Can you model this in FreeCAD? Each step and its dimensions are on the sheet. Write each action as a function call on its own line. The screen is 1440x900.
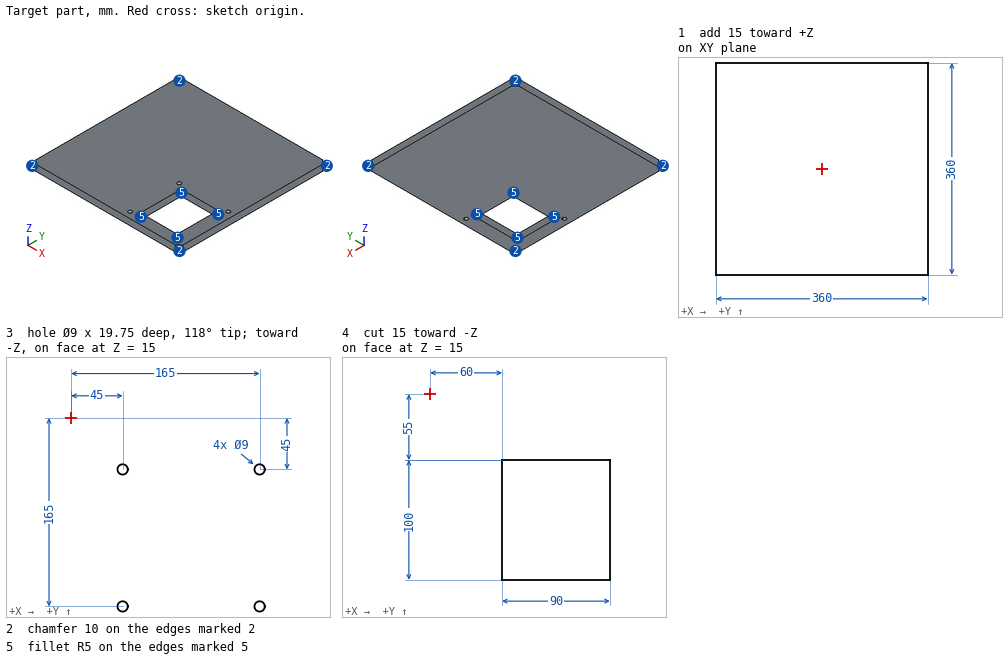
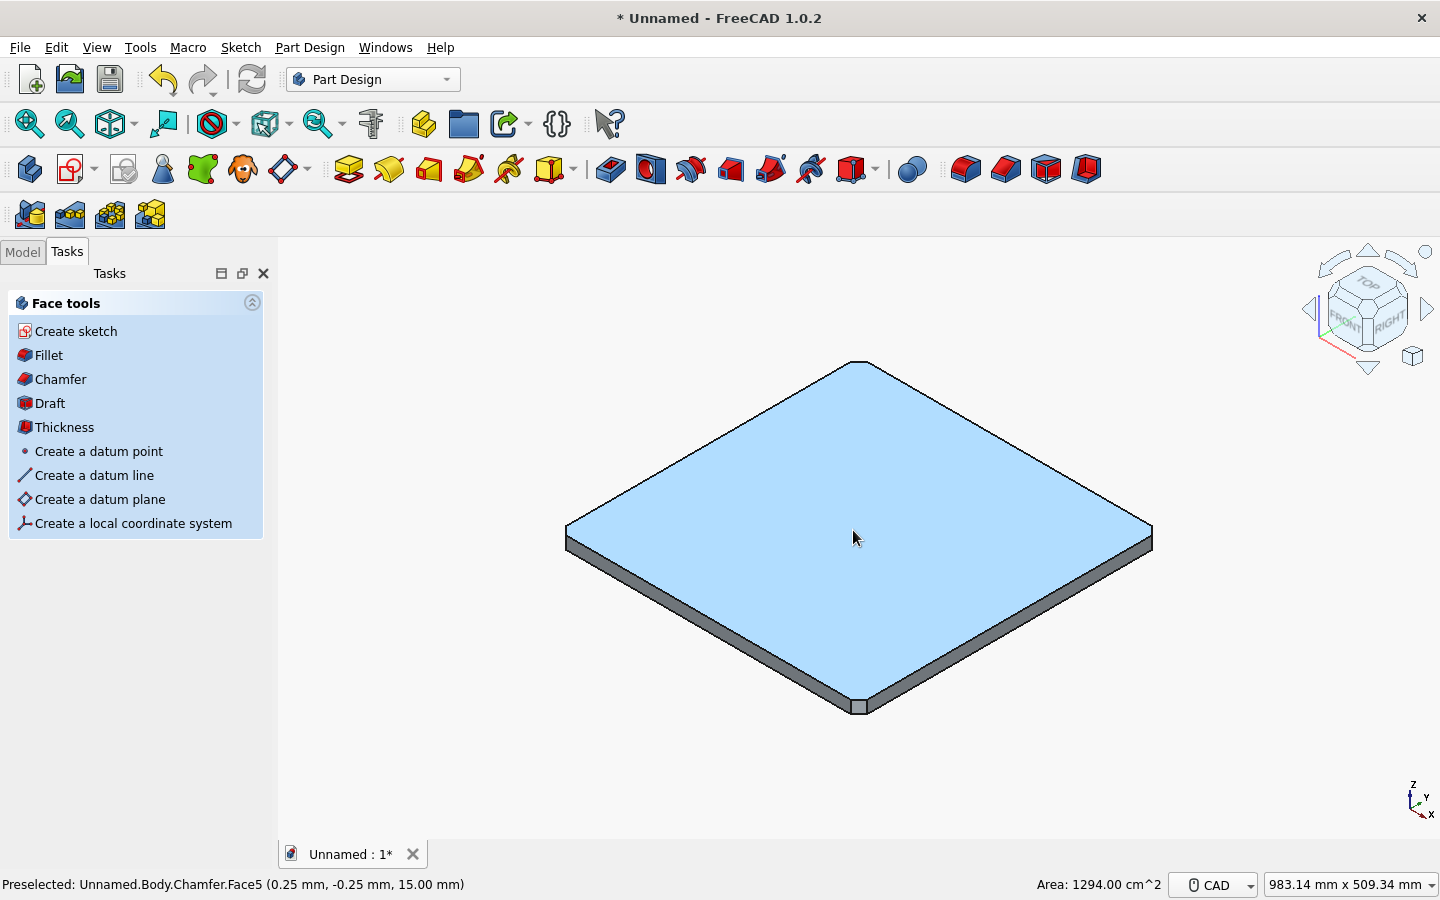
click(70, 170)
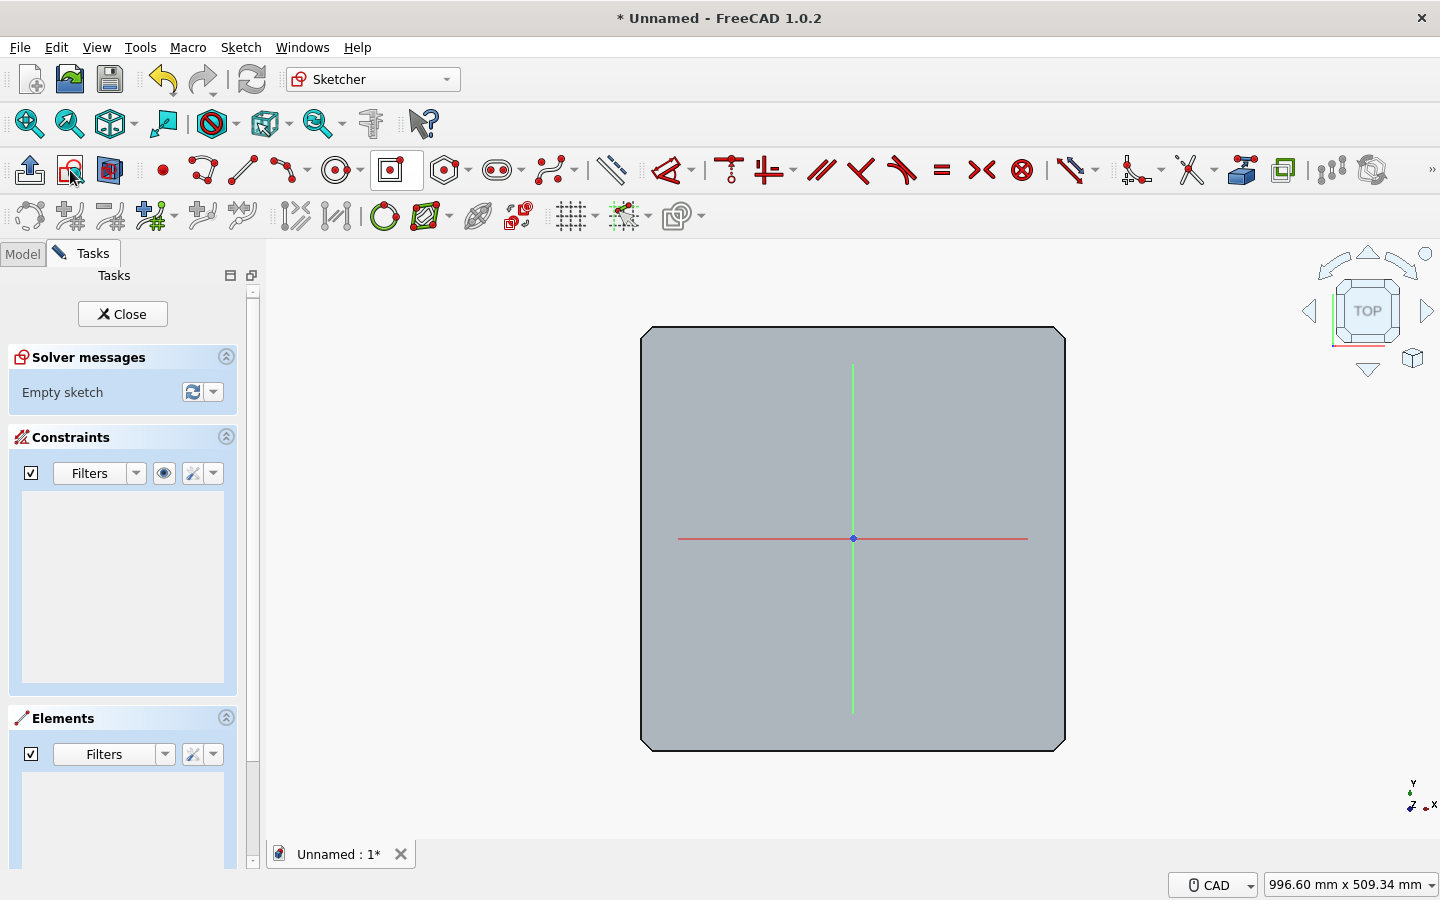
scroll(1158, 760, up, 3)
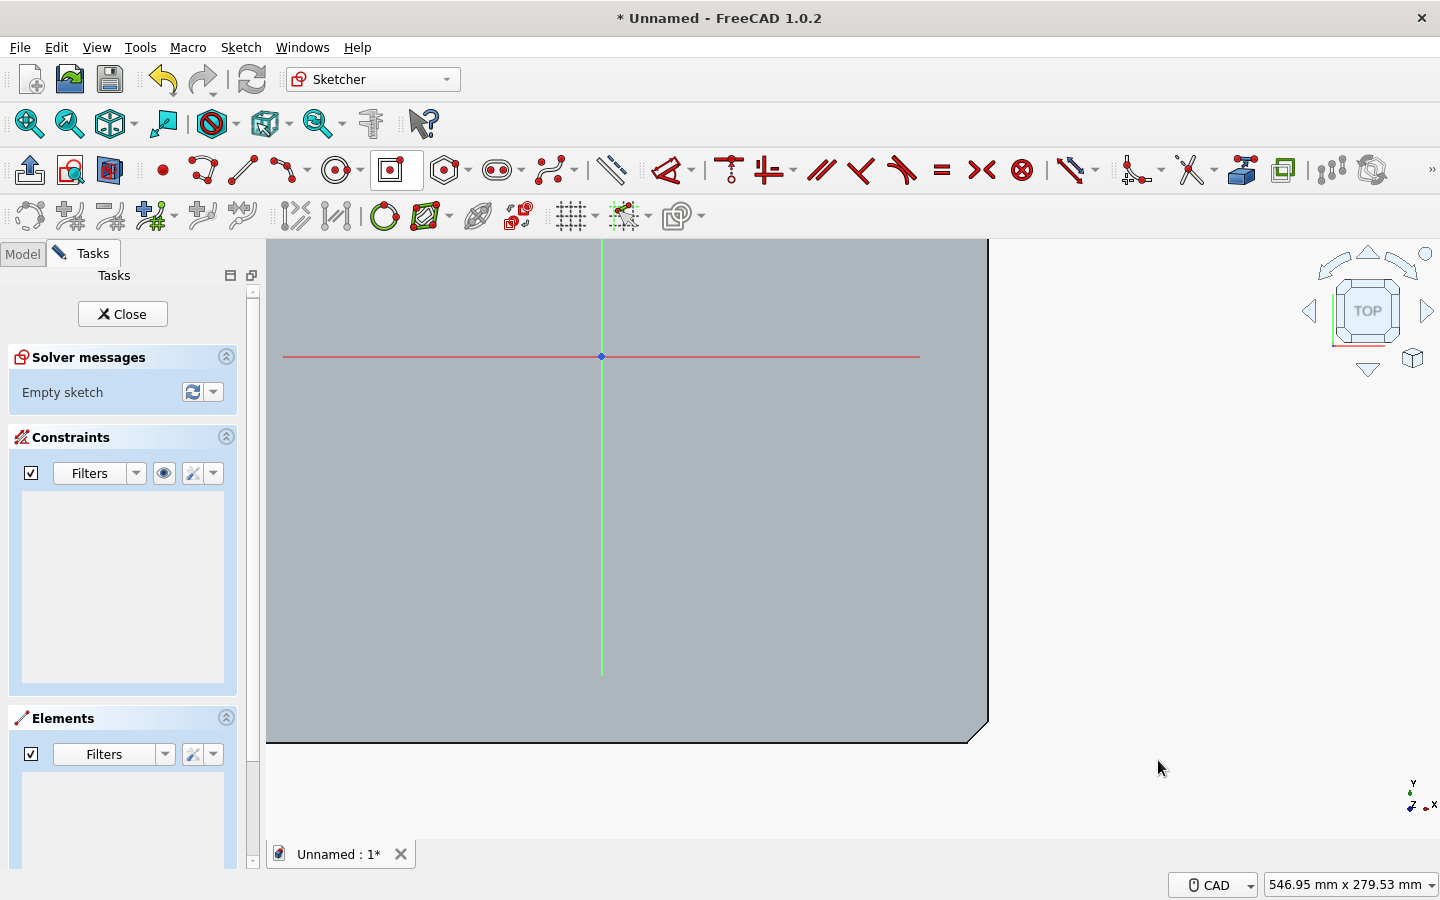
key(g)
key(c)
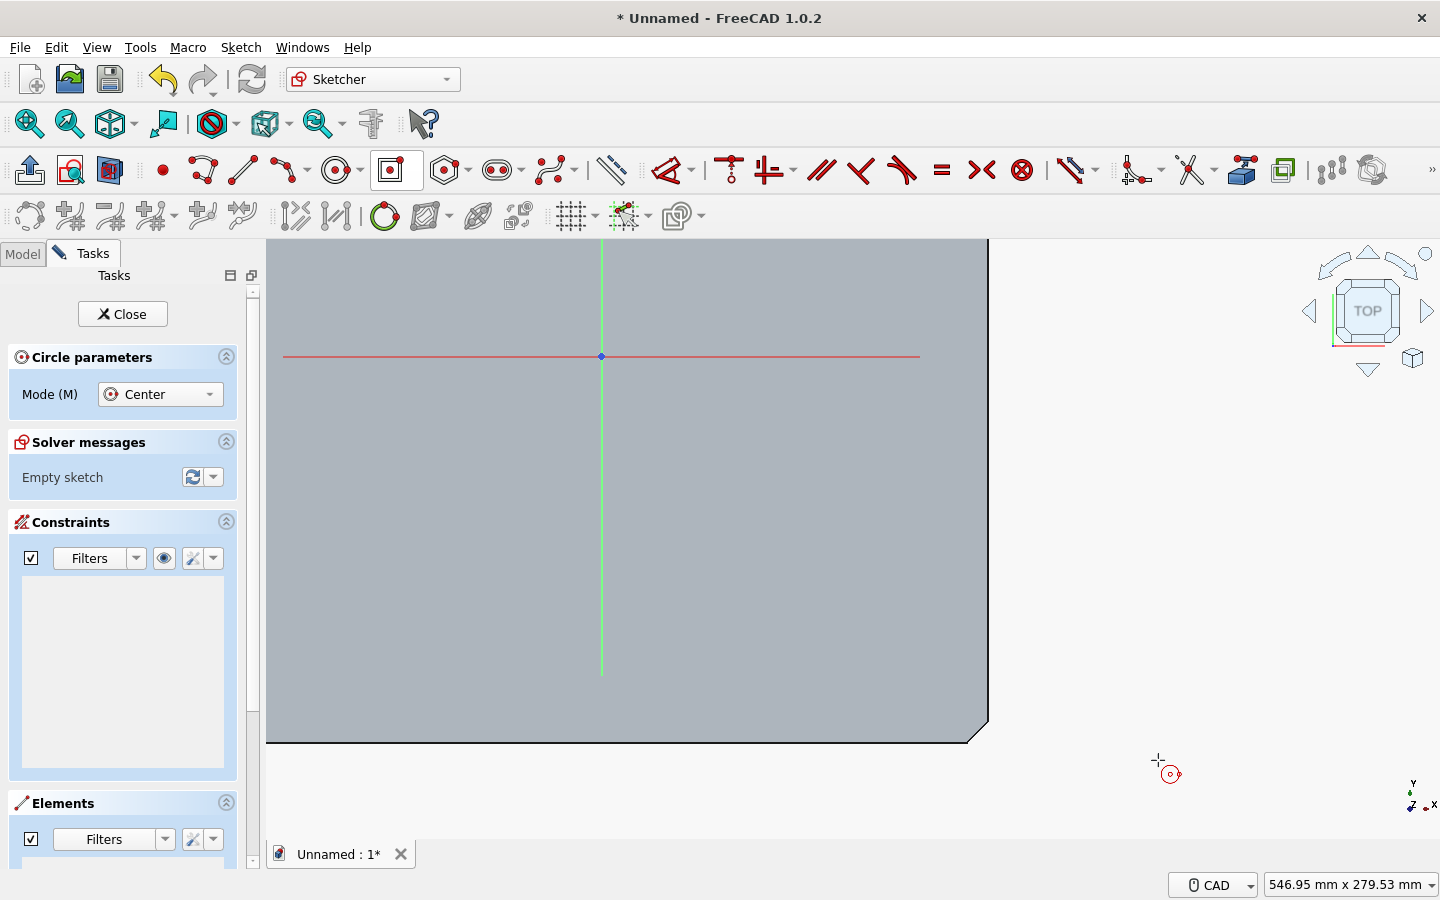
scroll(956, 453, up, 5)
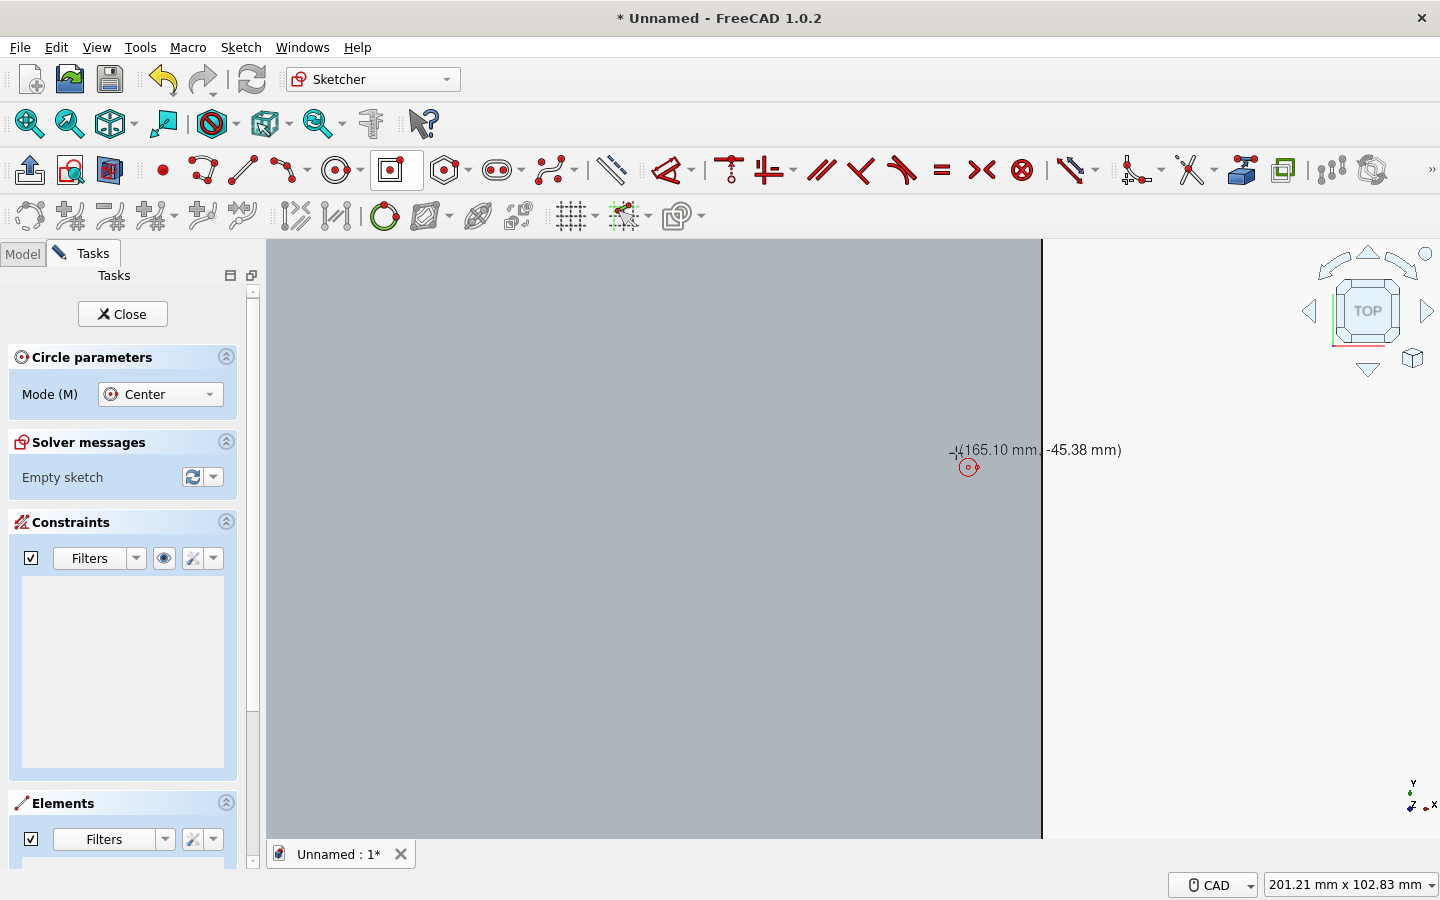
click(954, 453)
click(973, 434)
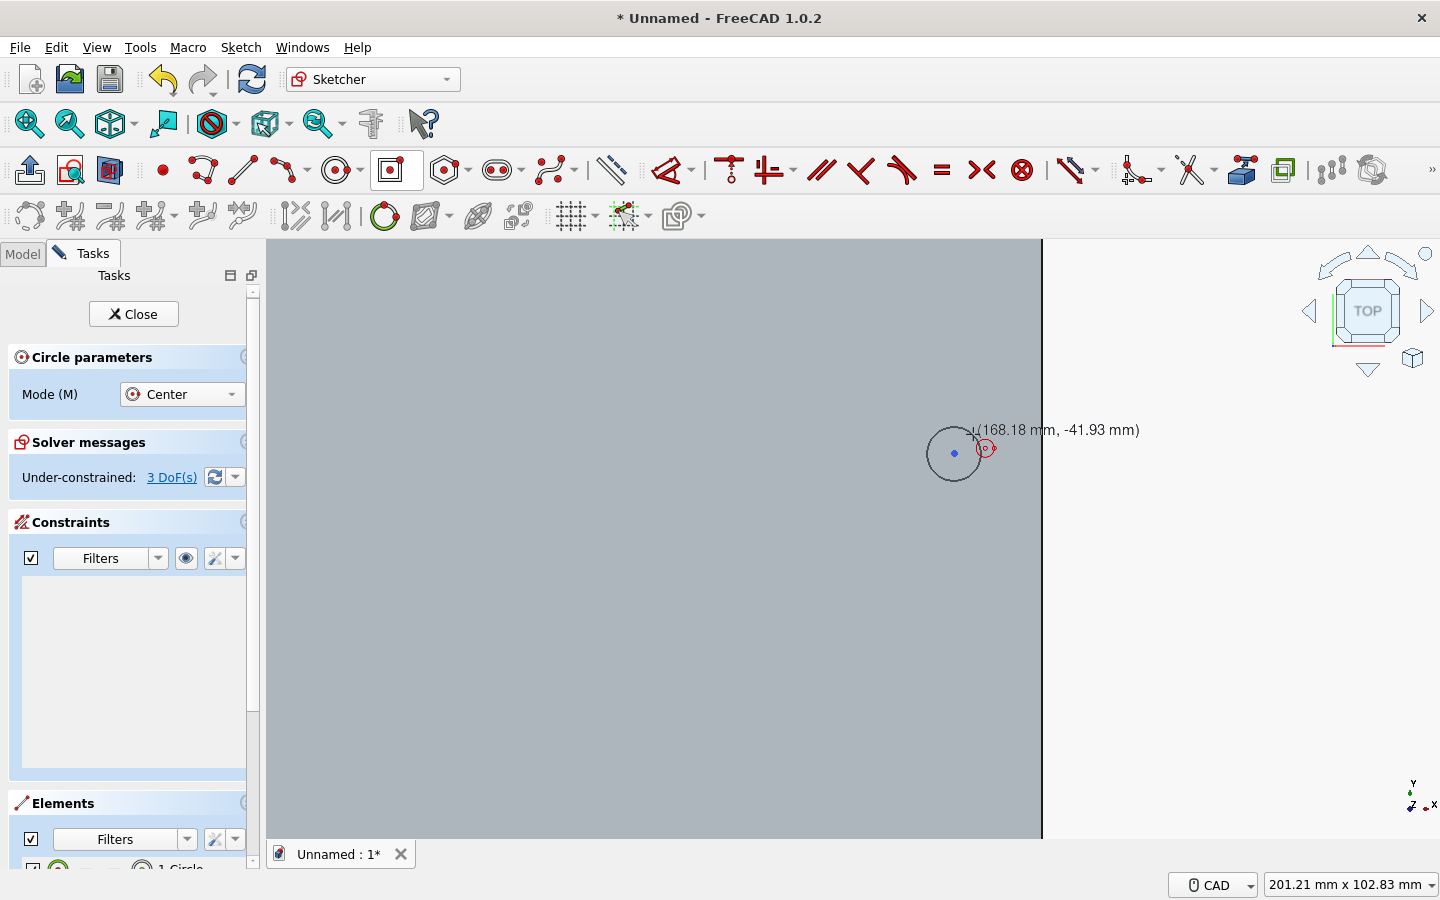
scroll(958, 454, down, 5)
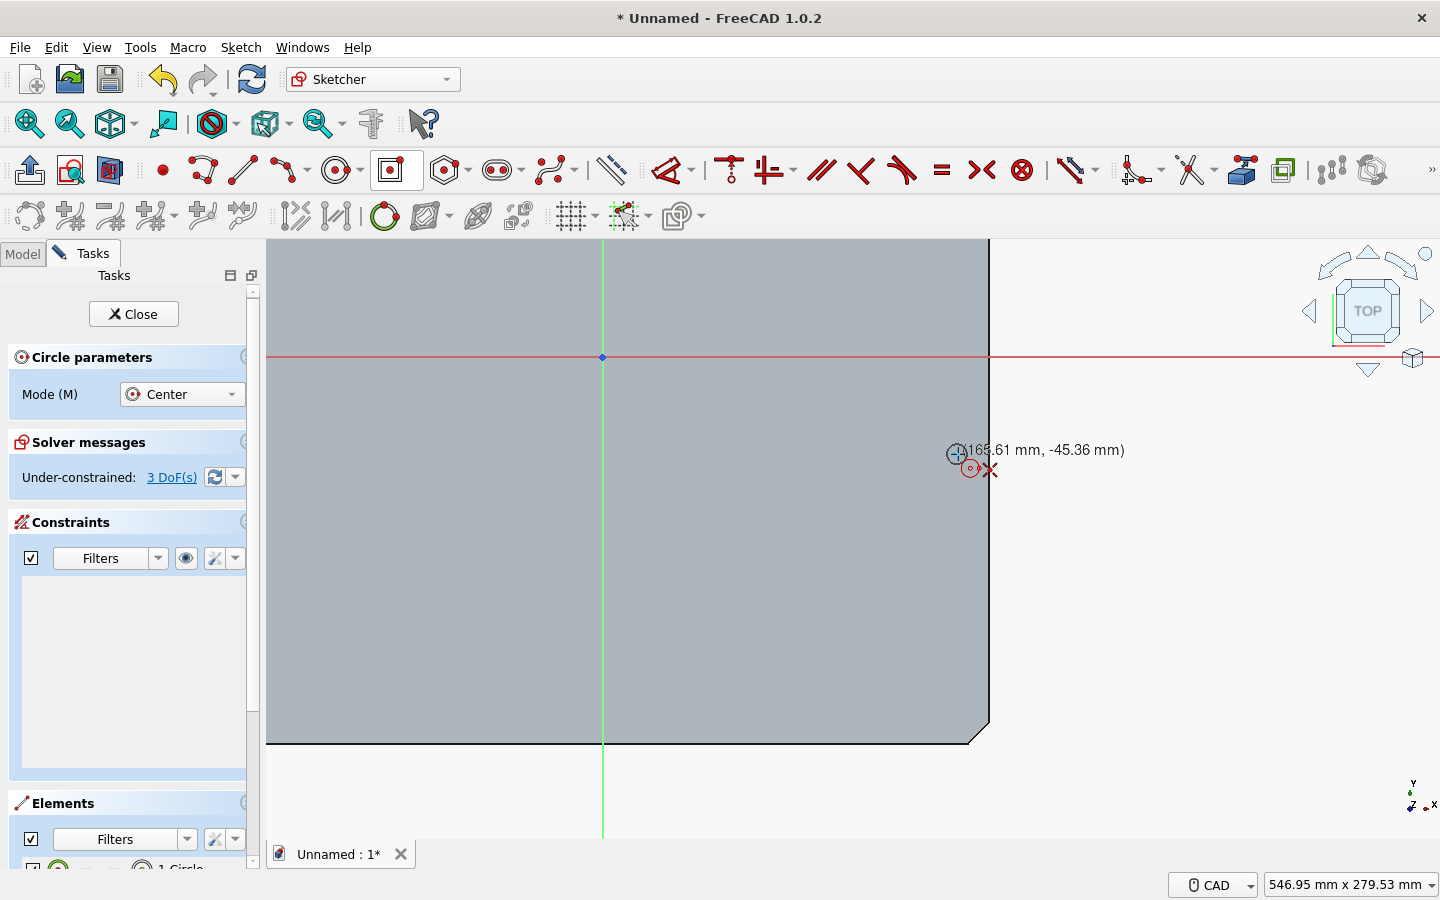
scroll(699, 454, up, 5)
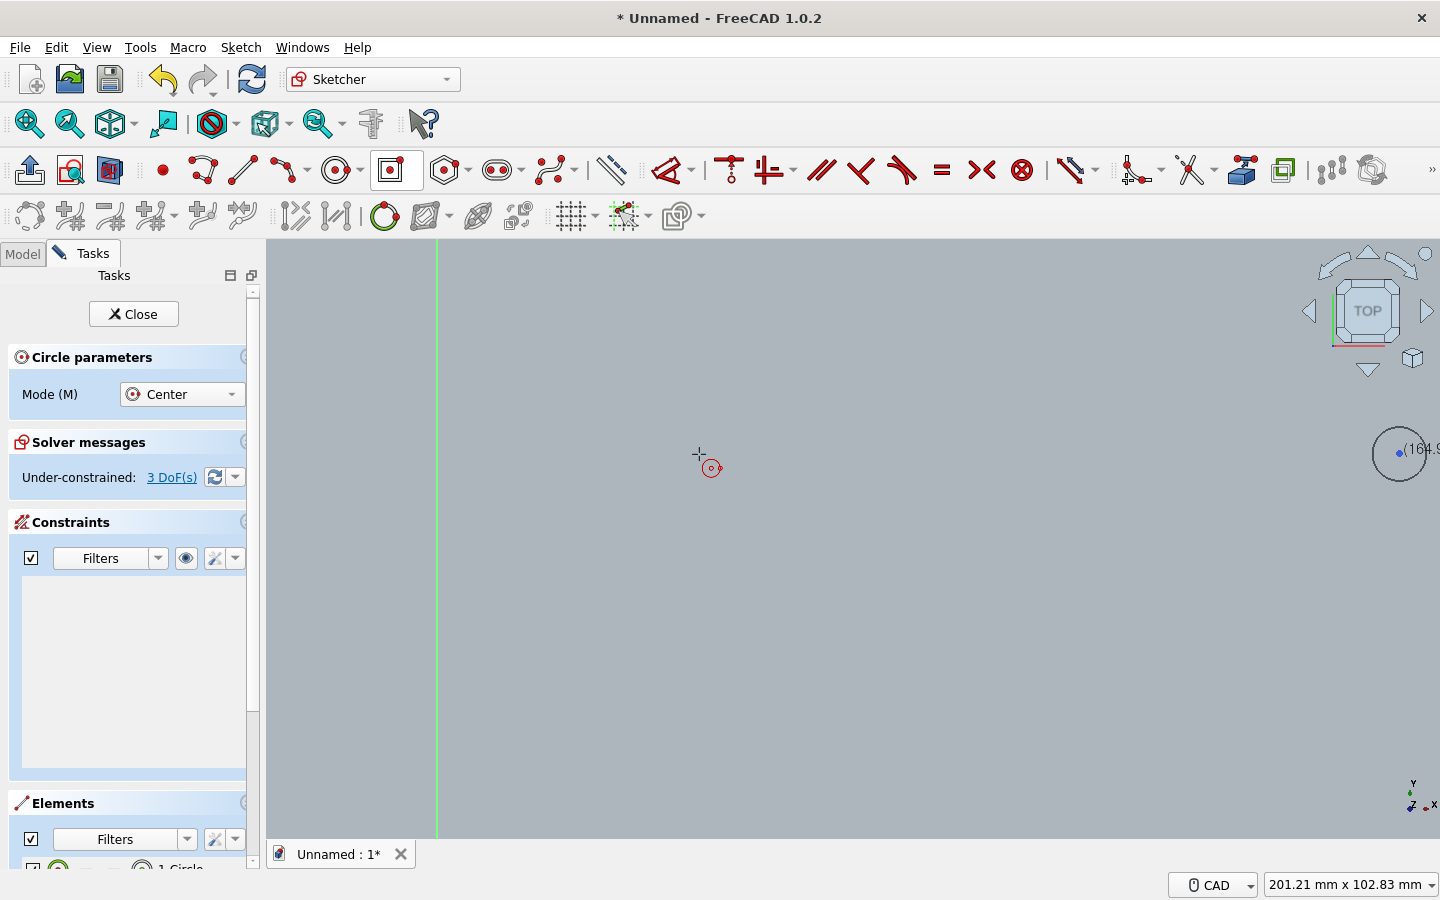
click(700, 453)
click(718, 434)